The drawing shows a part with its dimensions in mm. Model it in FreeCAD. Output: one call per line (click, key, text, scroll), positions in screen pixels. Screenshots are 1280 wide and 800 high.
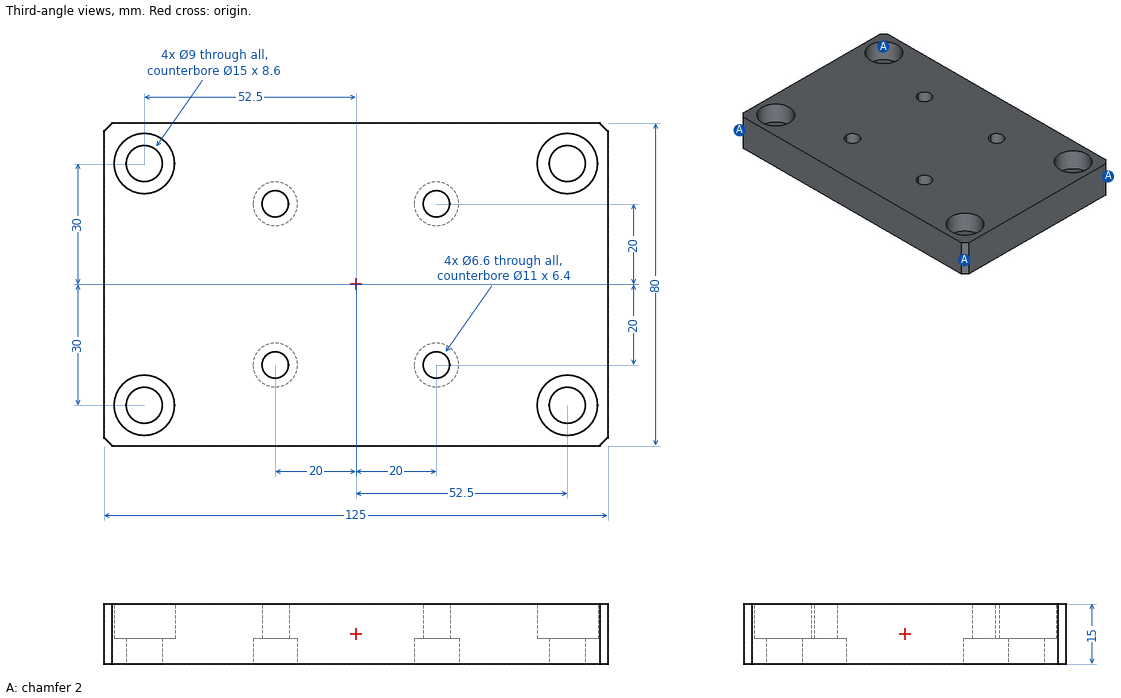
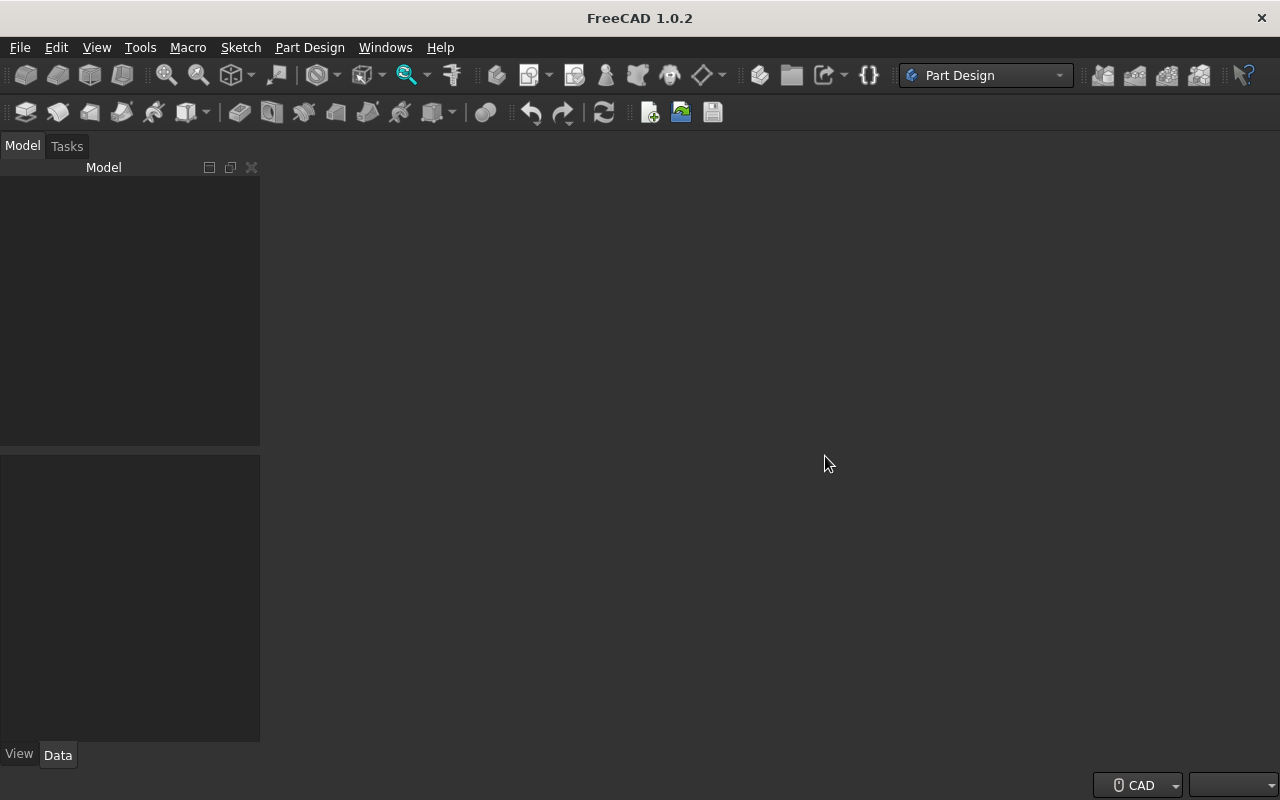
key(ctrl+n)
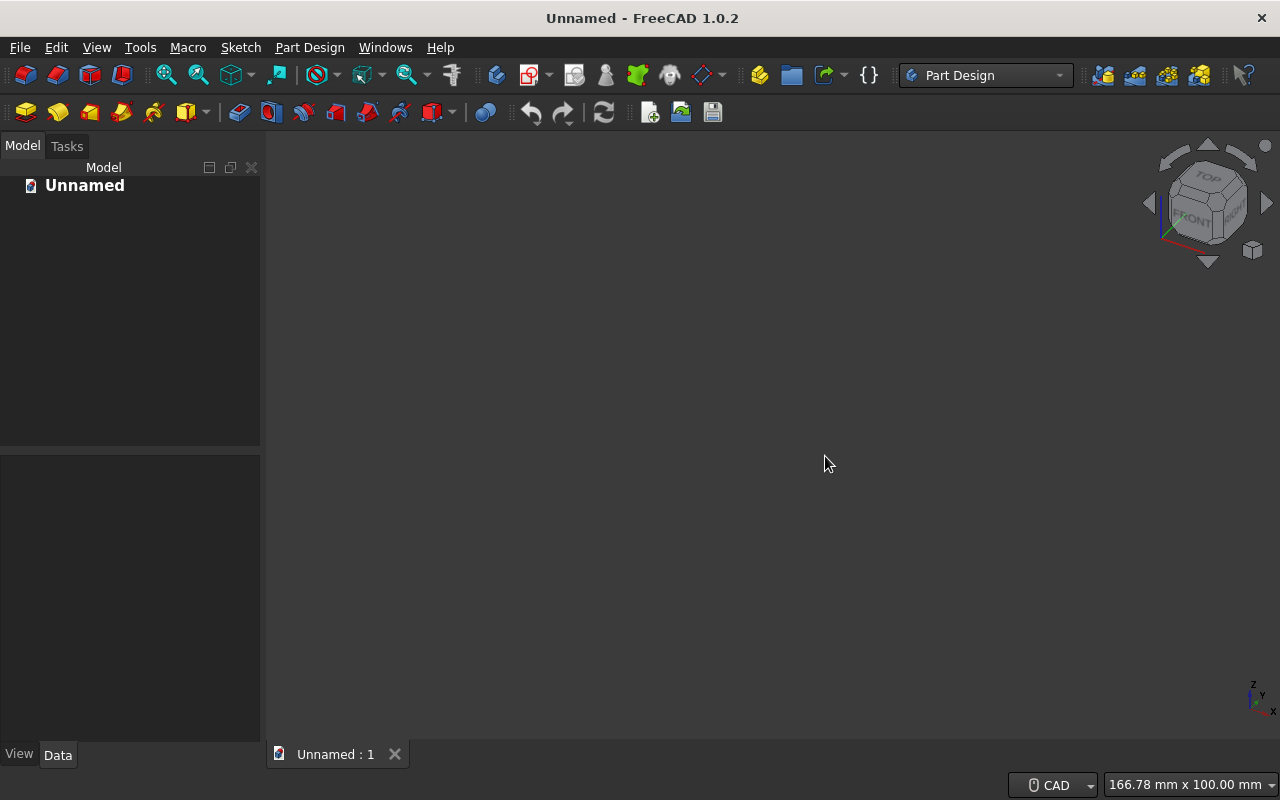
click(530, 76)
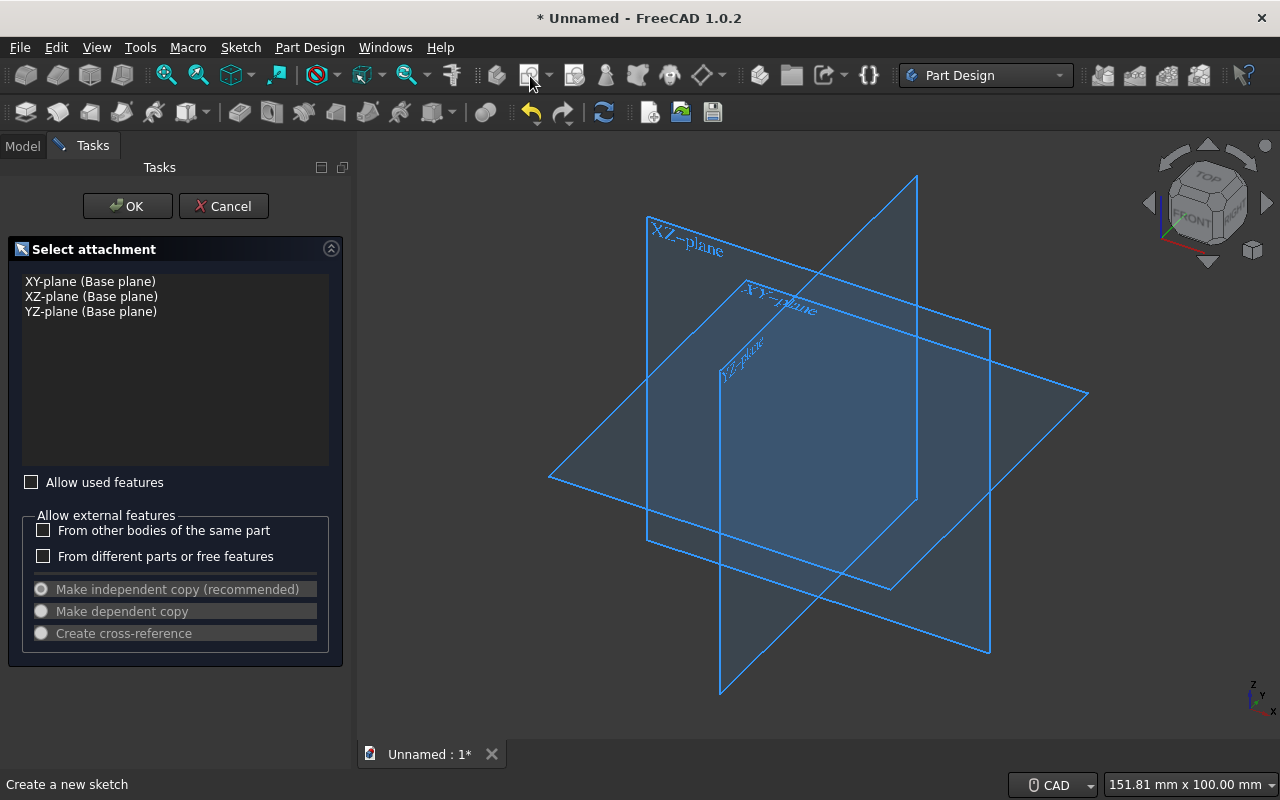
click(82, 282)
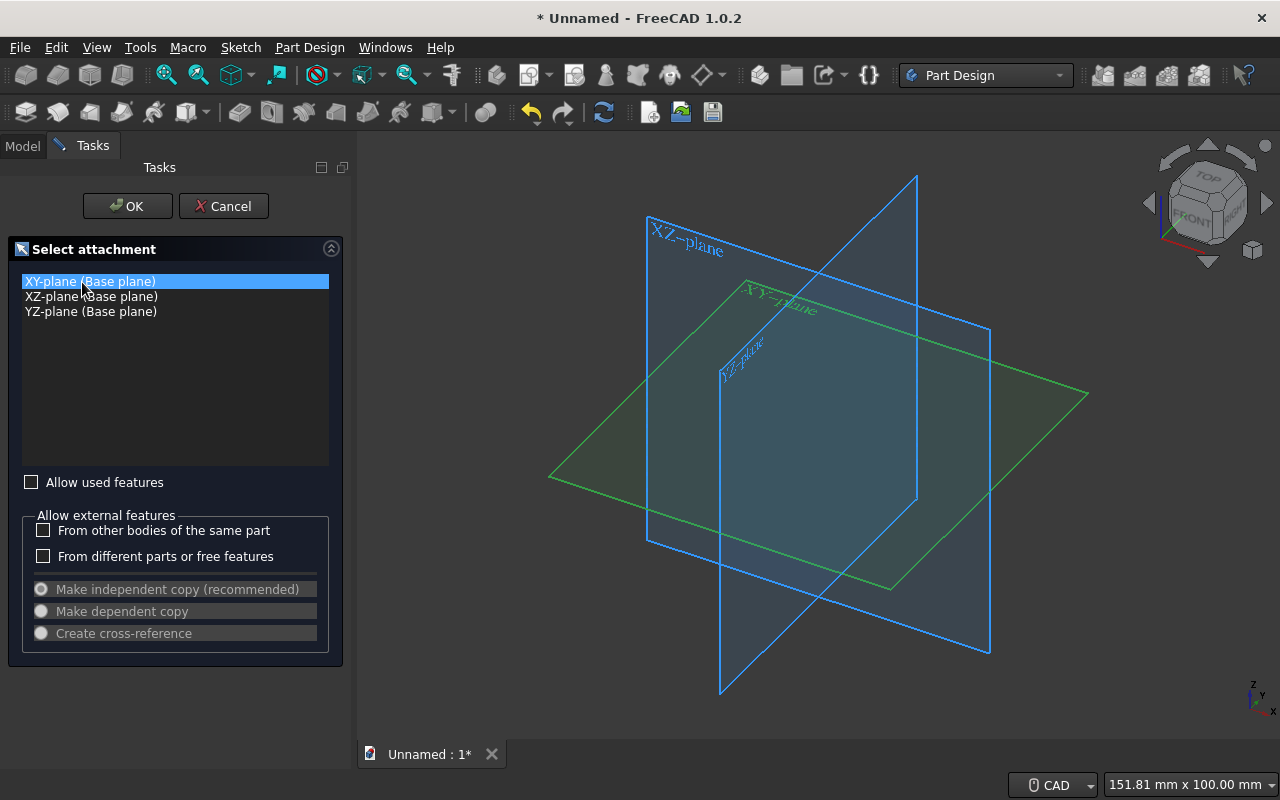
click(128, 206)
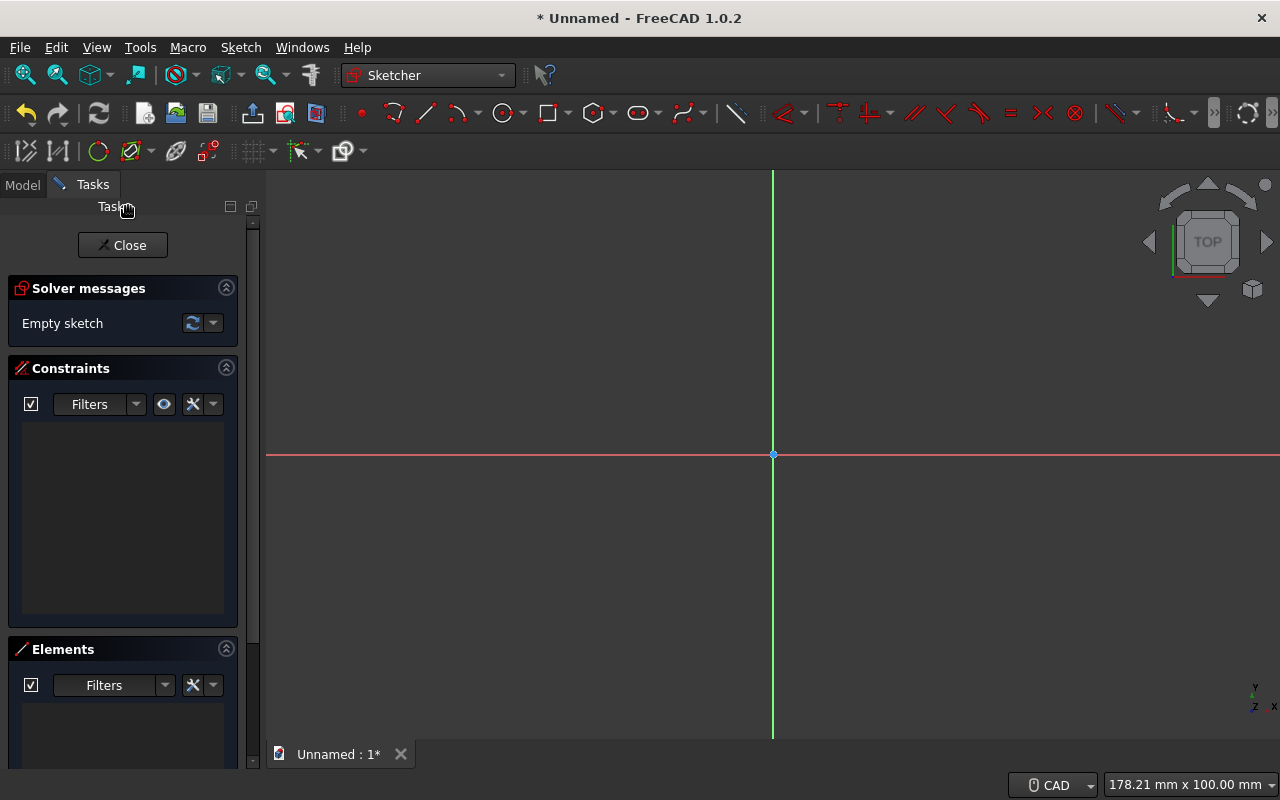
scroll(395, 455, down, 1)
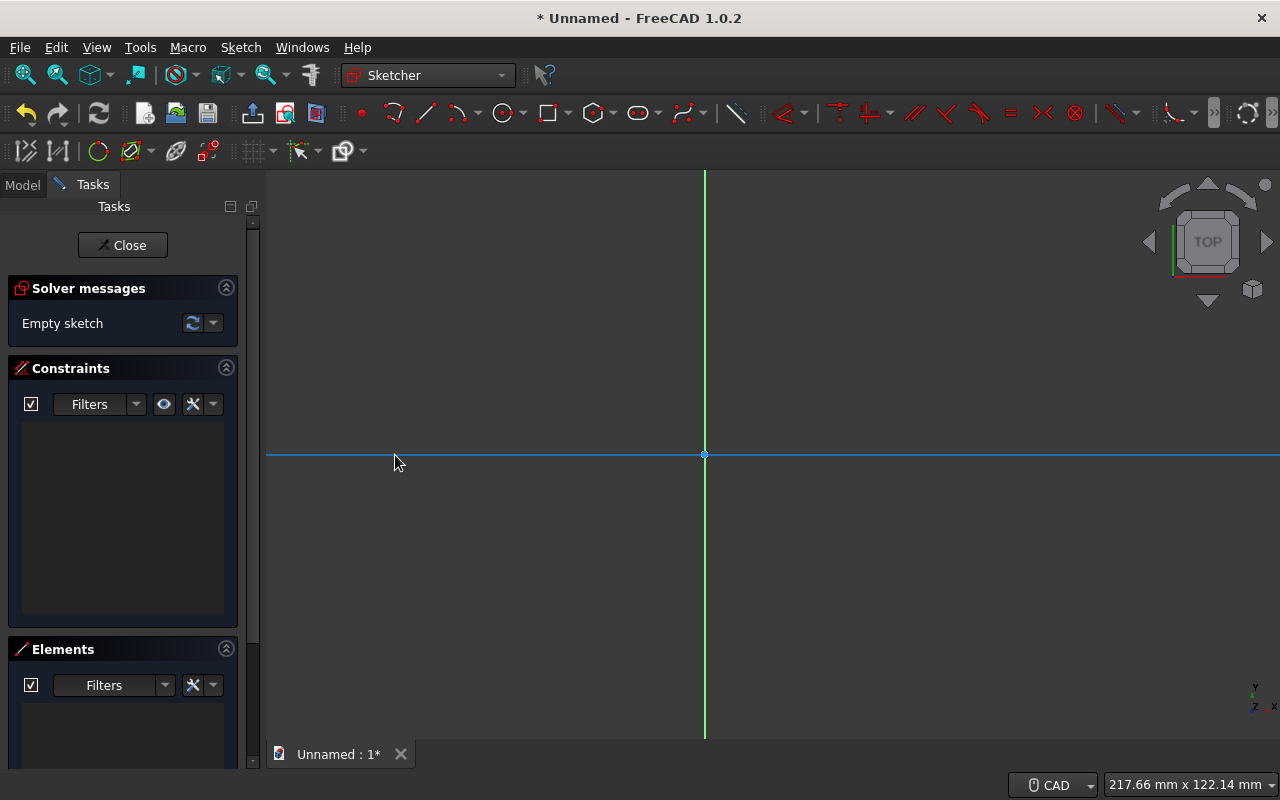
key(g)
key(v)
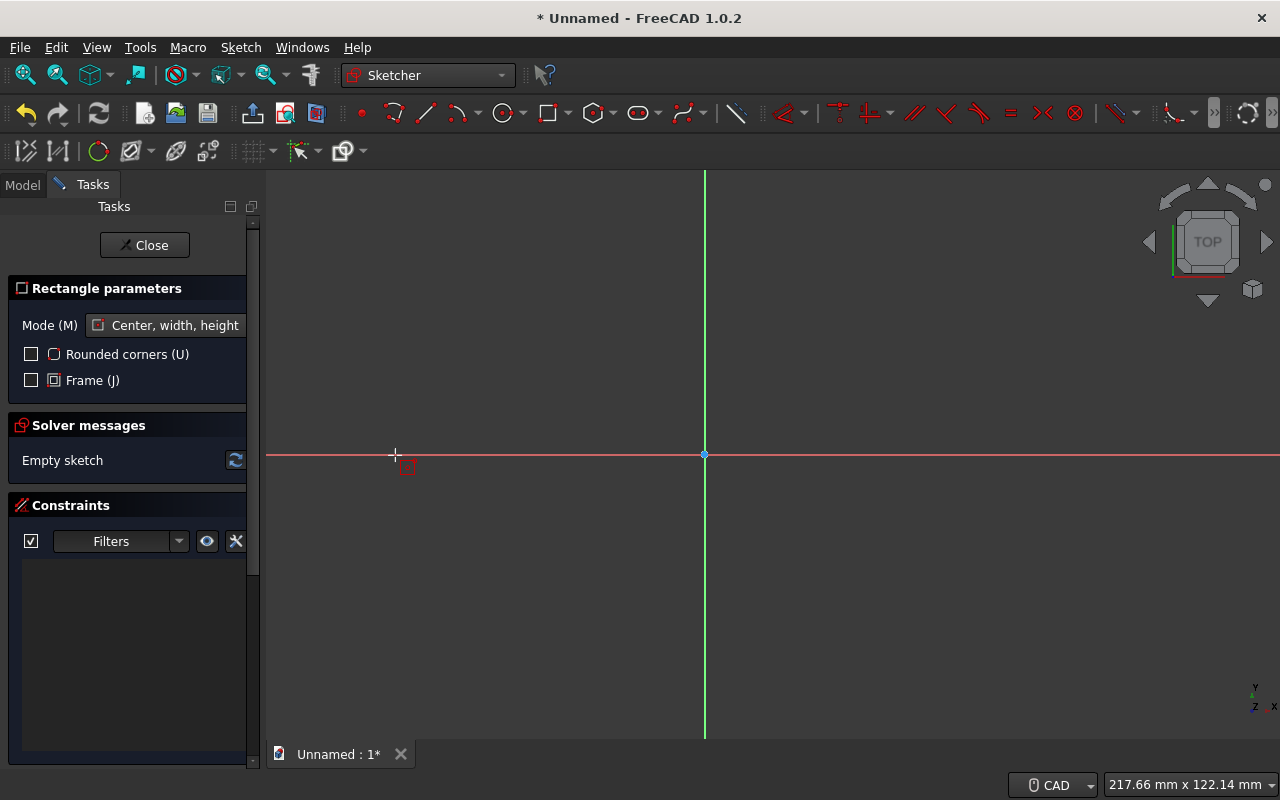
click(705, 455)
move(996, 268)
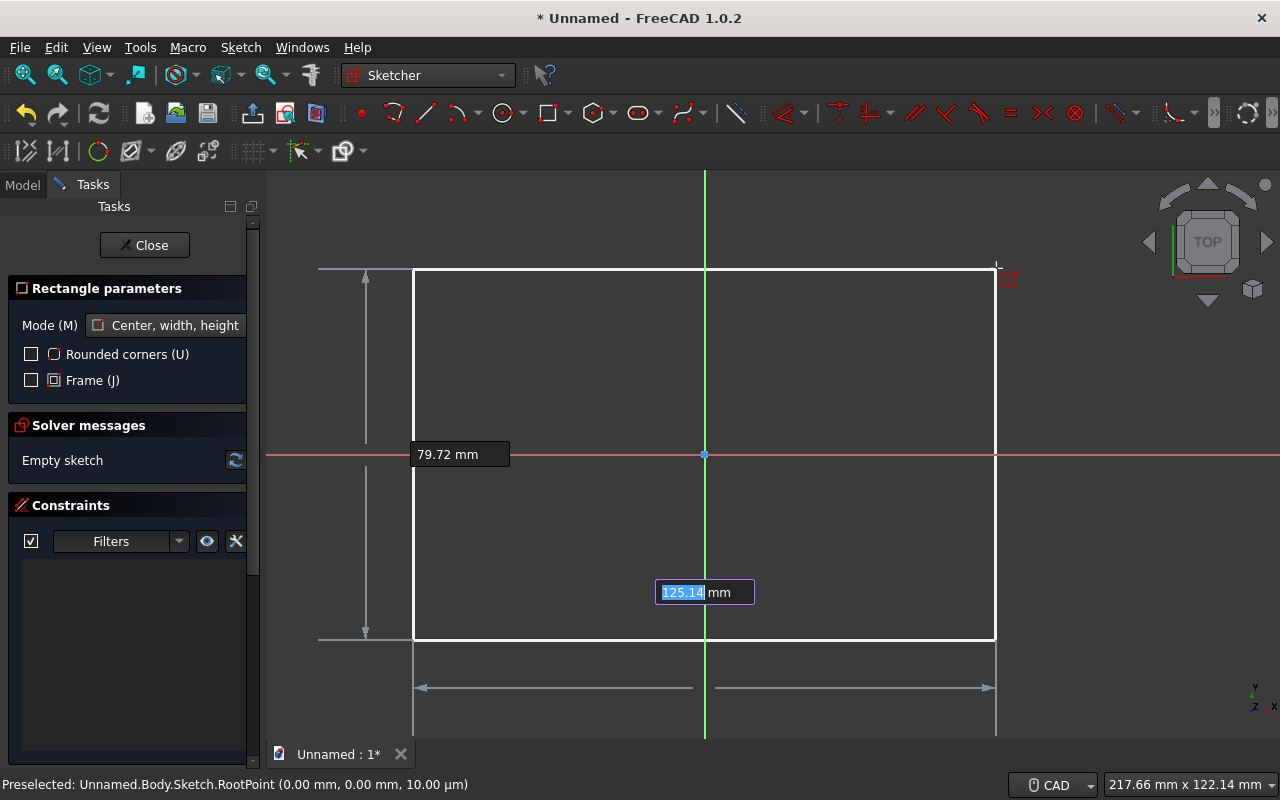
text(125)
key(Tab)
text(80)
key(Return)
key(Escape)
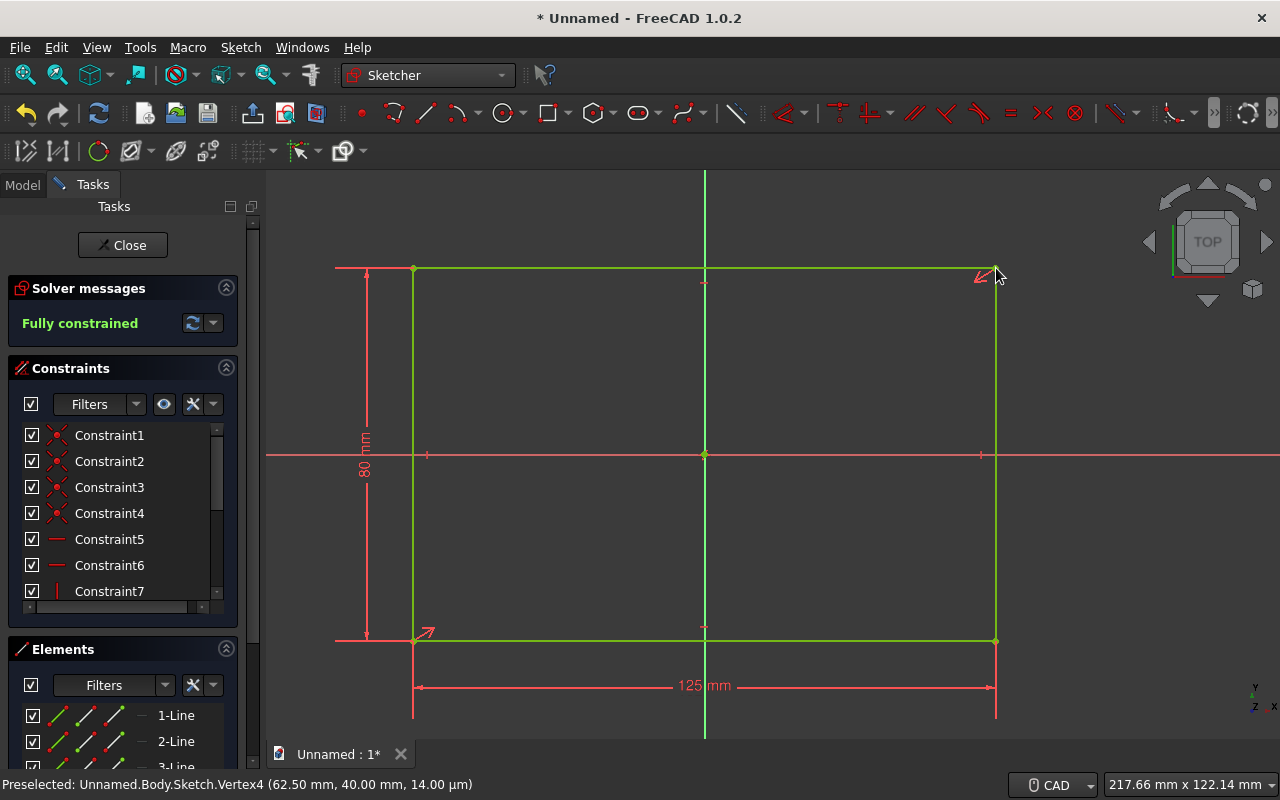
click(123, 245)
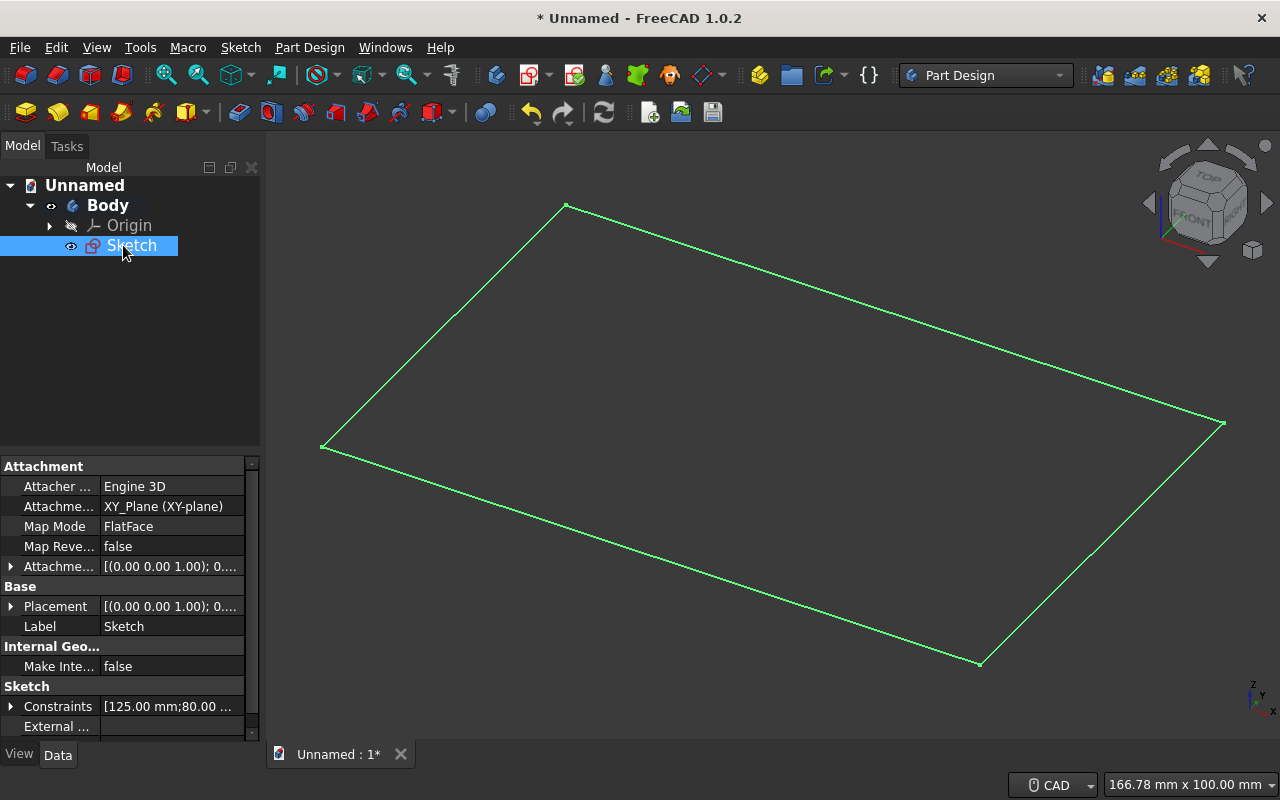
click(26, 112)